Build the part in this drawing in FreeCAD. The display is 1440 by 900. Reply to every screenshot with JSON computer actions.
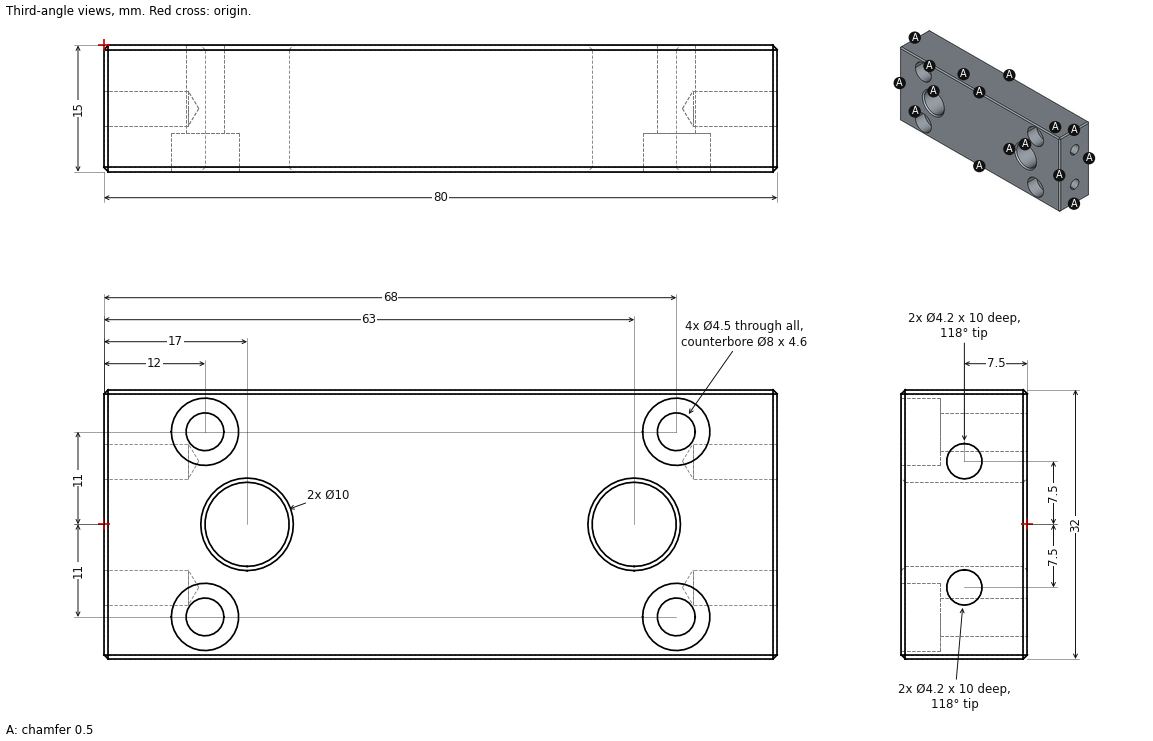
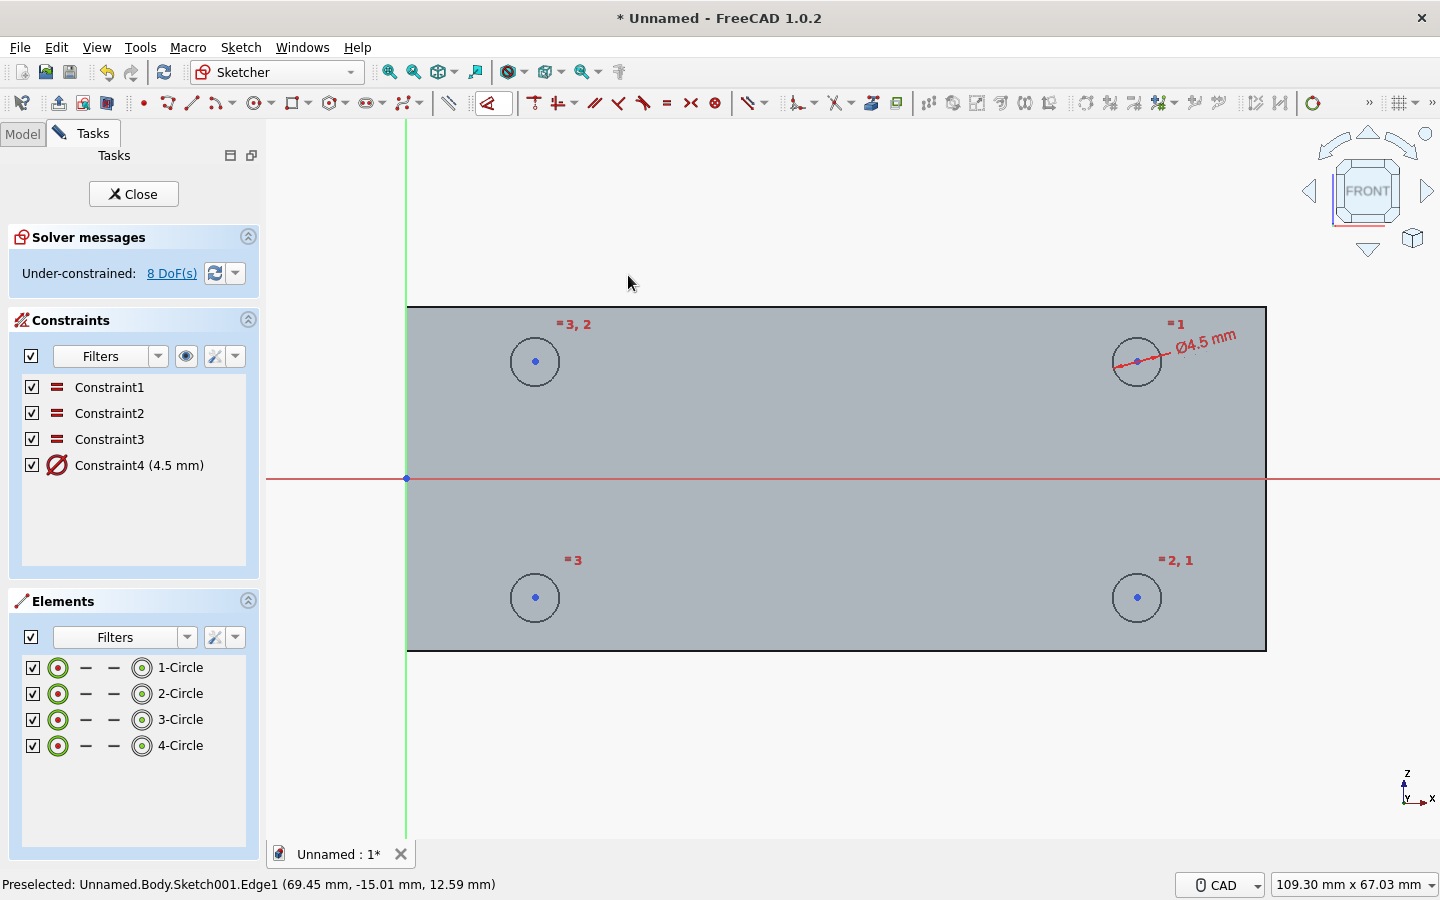
{"action": "left_click", "coordinate": [1137, 362]}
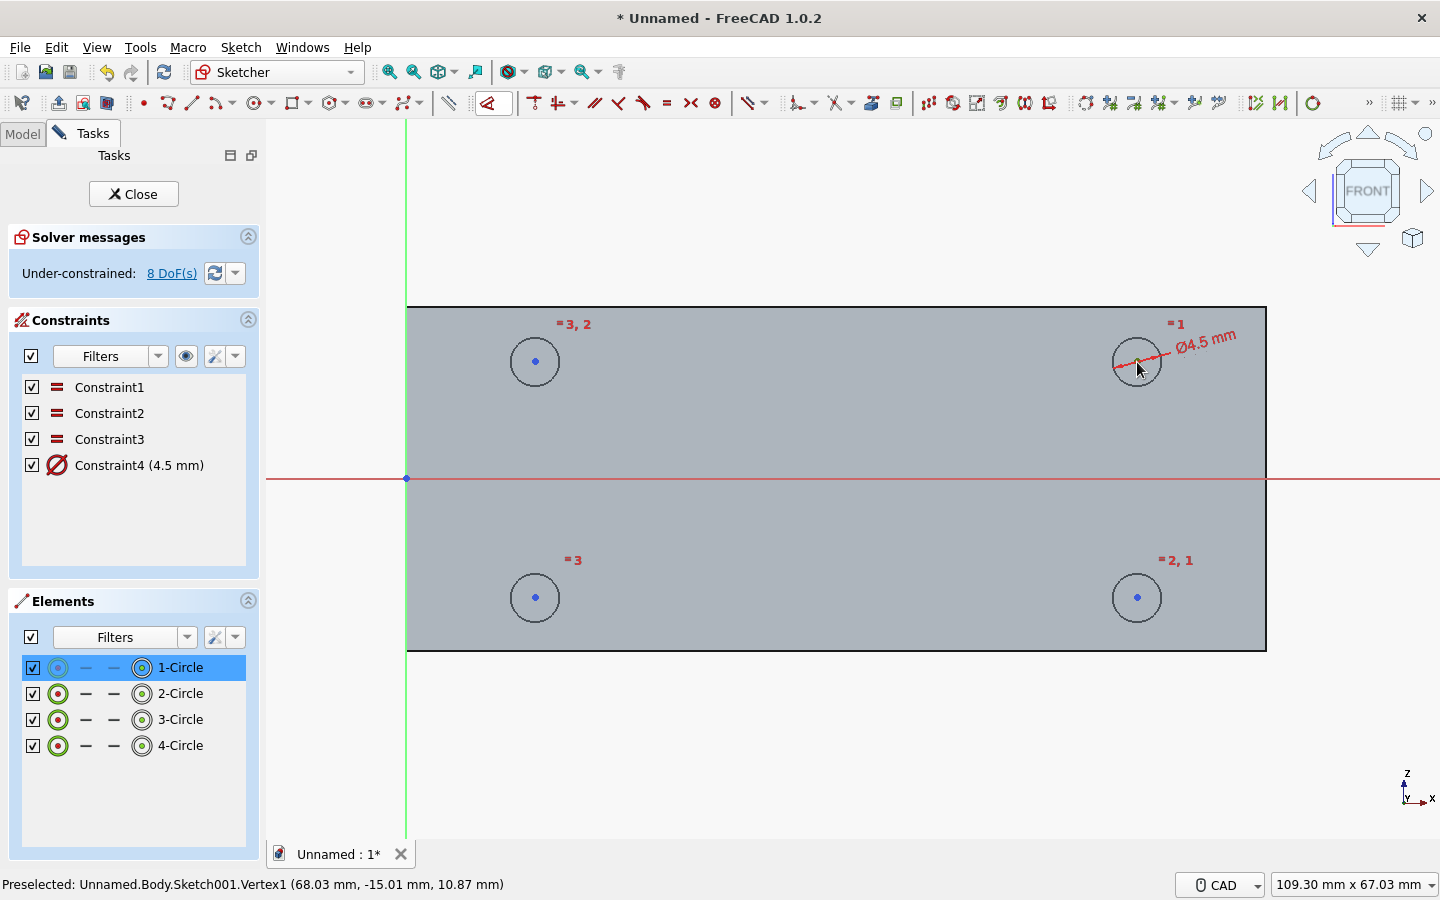
{"action": "key", "text": "l"}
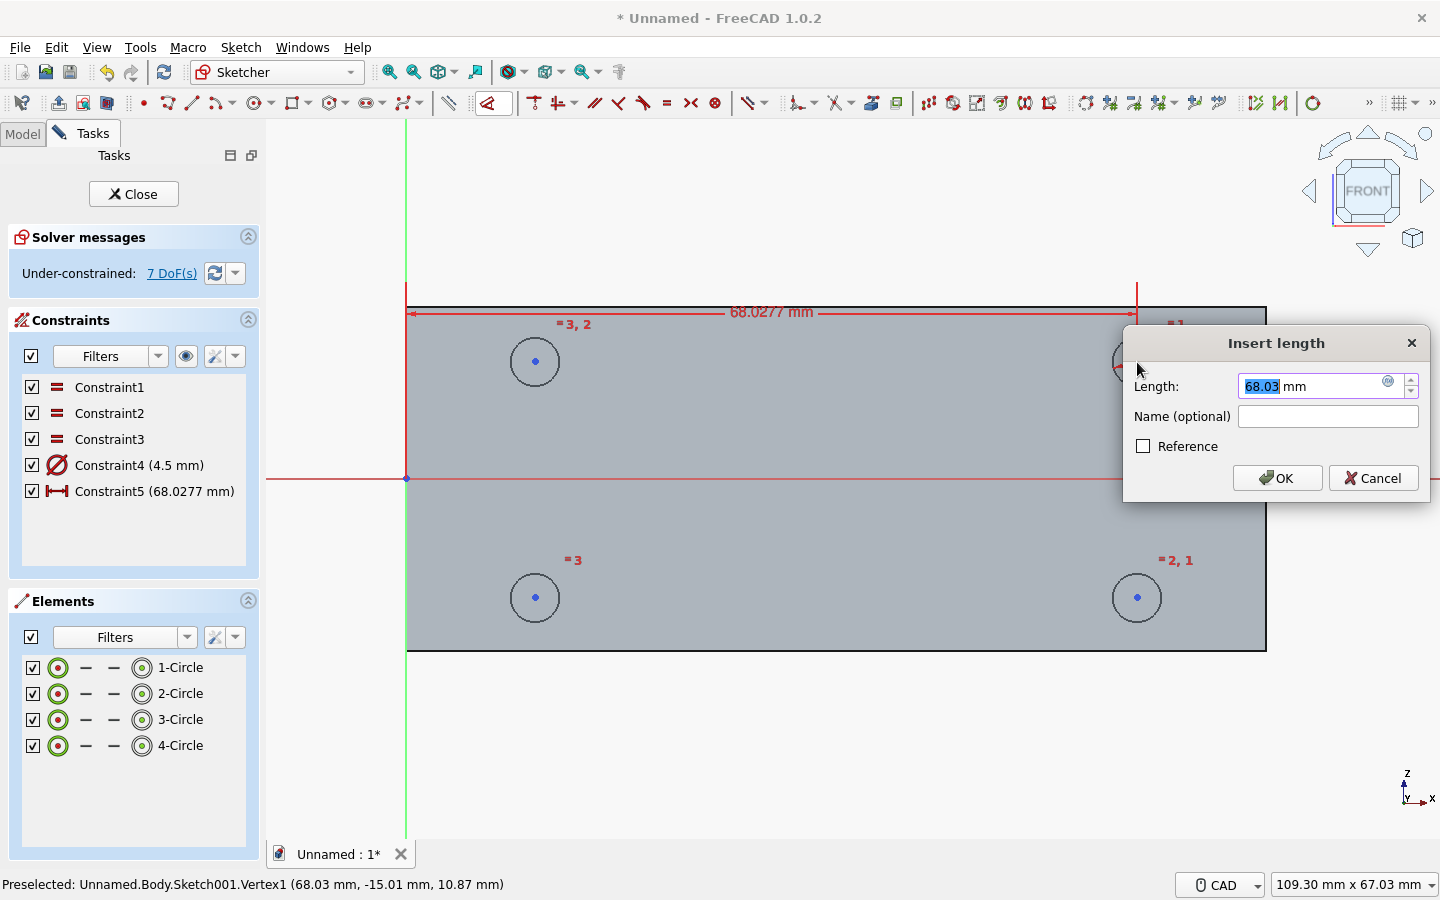
{"action": "type", "text": "68"}
{"action": "key", "text": "Return"}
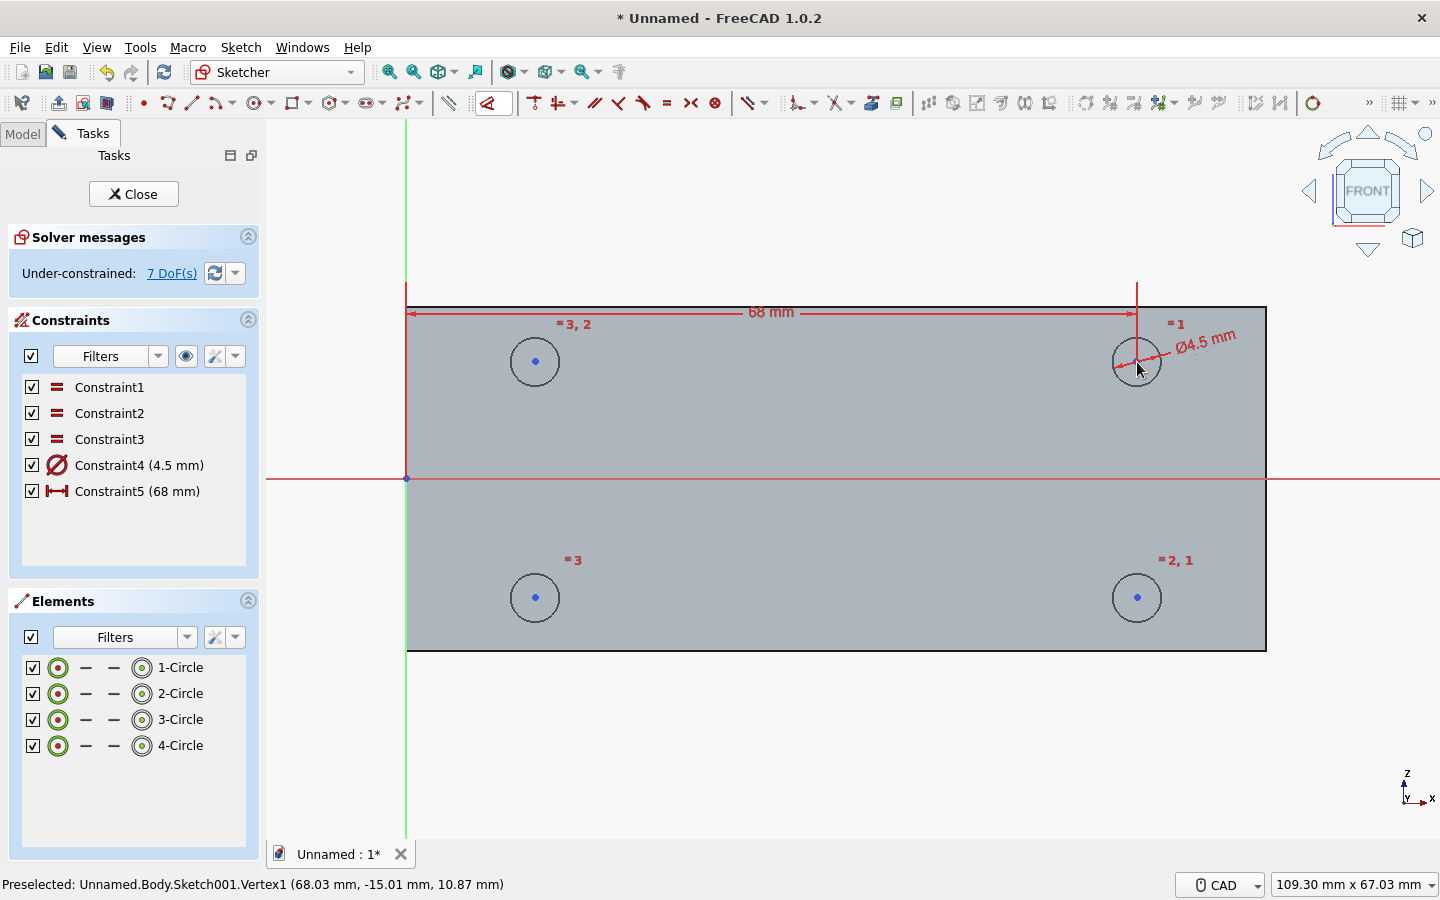
{"action": "left_click", "coordinate": [1137, 362]}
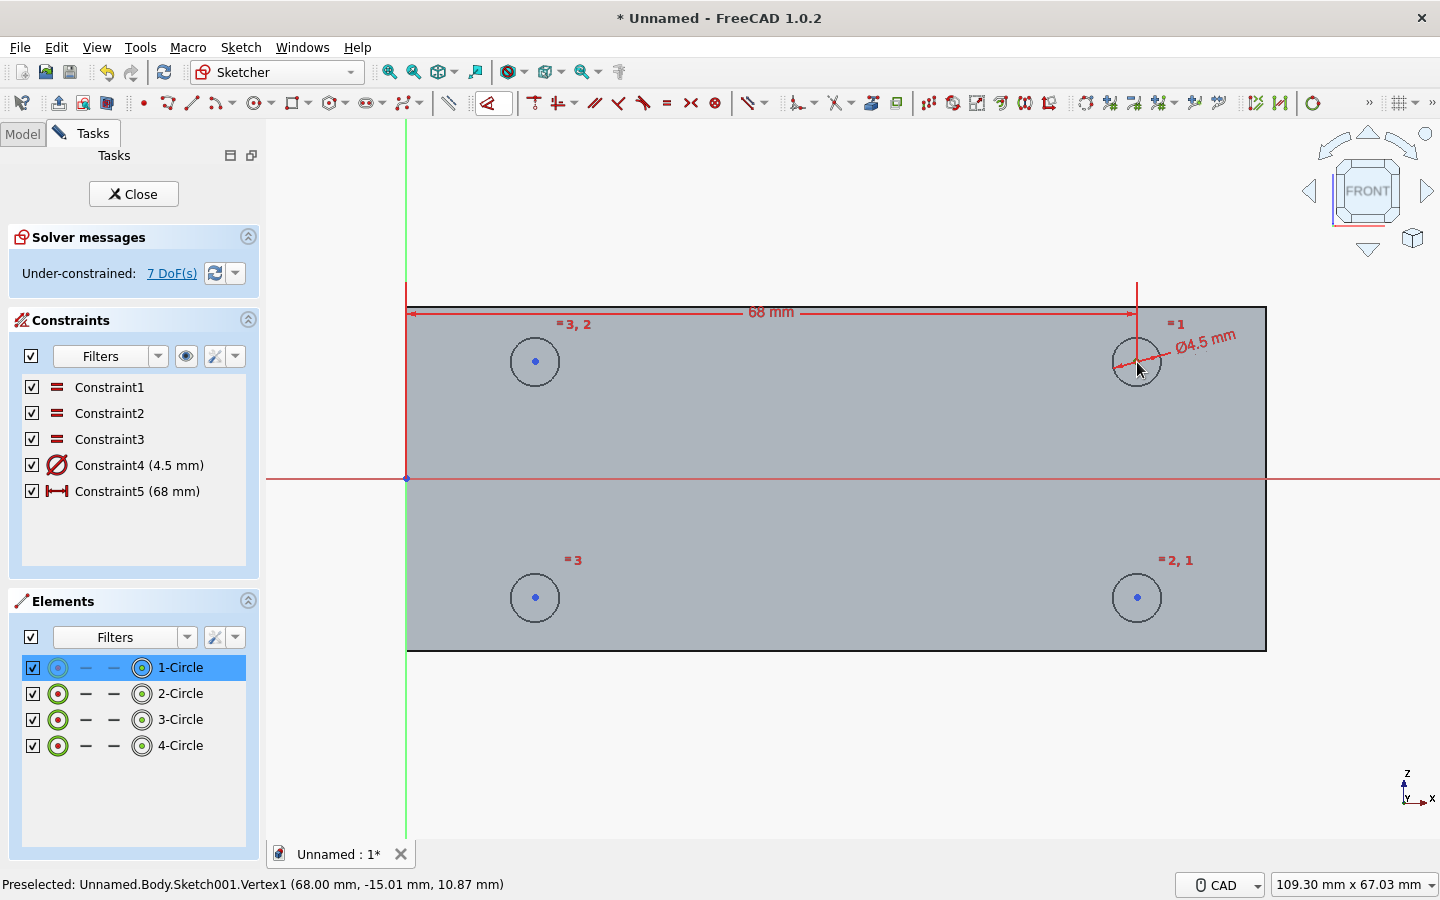
{"action": "key", "text": "i"}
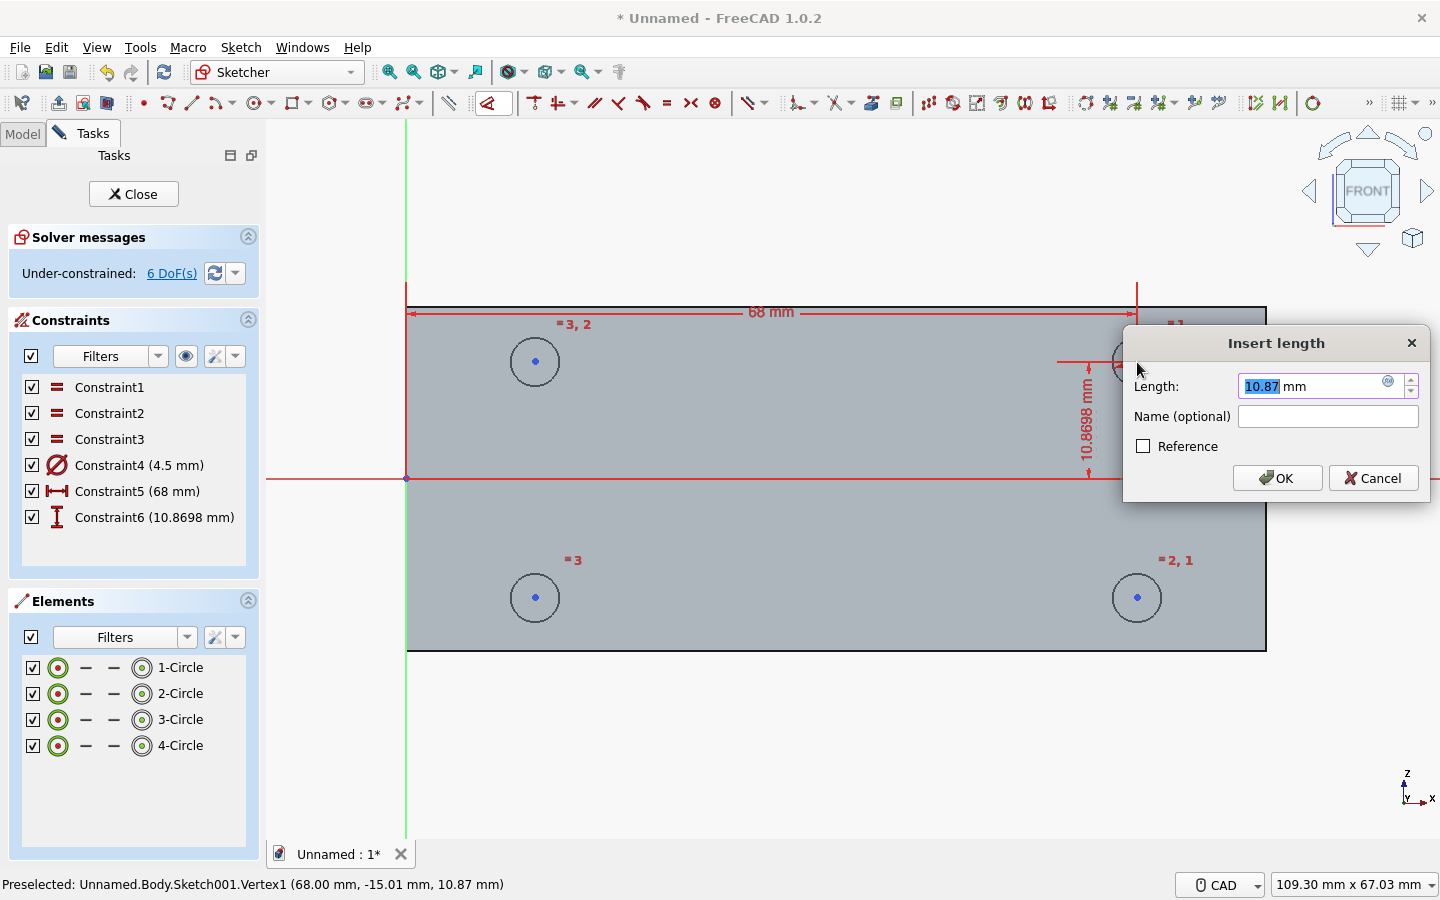
{"action": "type", "text": "11"}
{"action": "key", "text": "Return"}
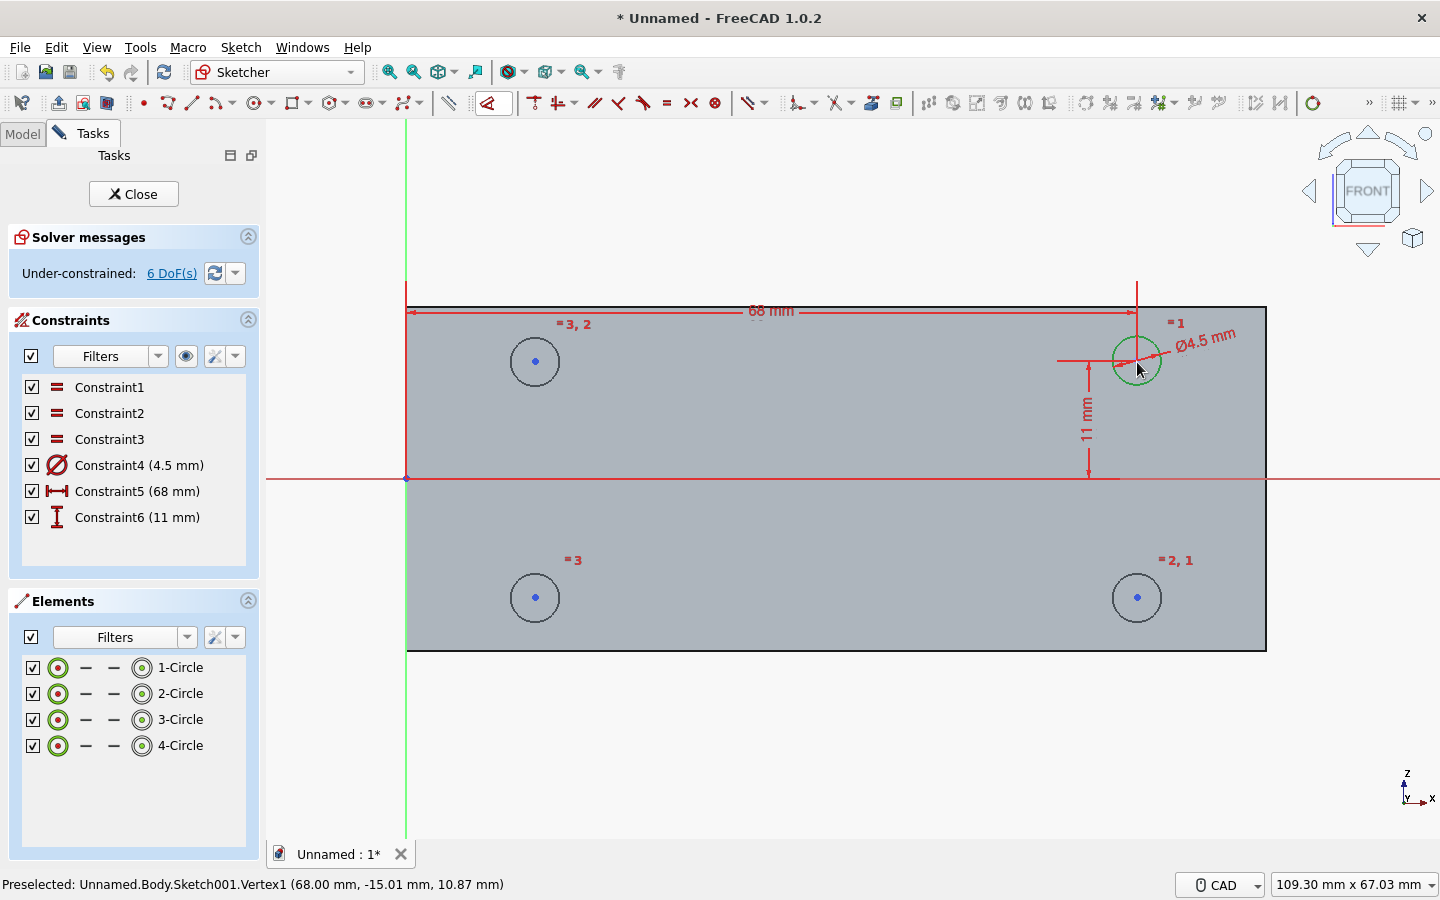
{"action": "left_click", "coordinate": [1137, 598]}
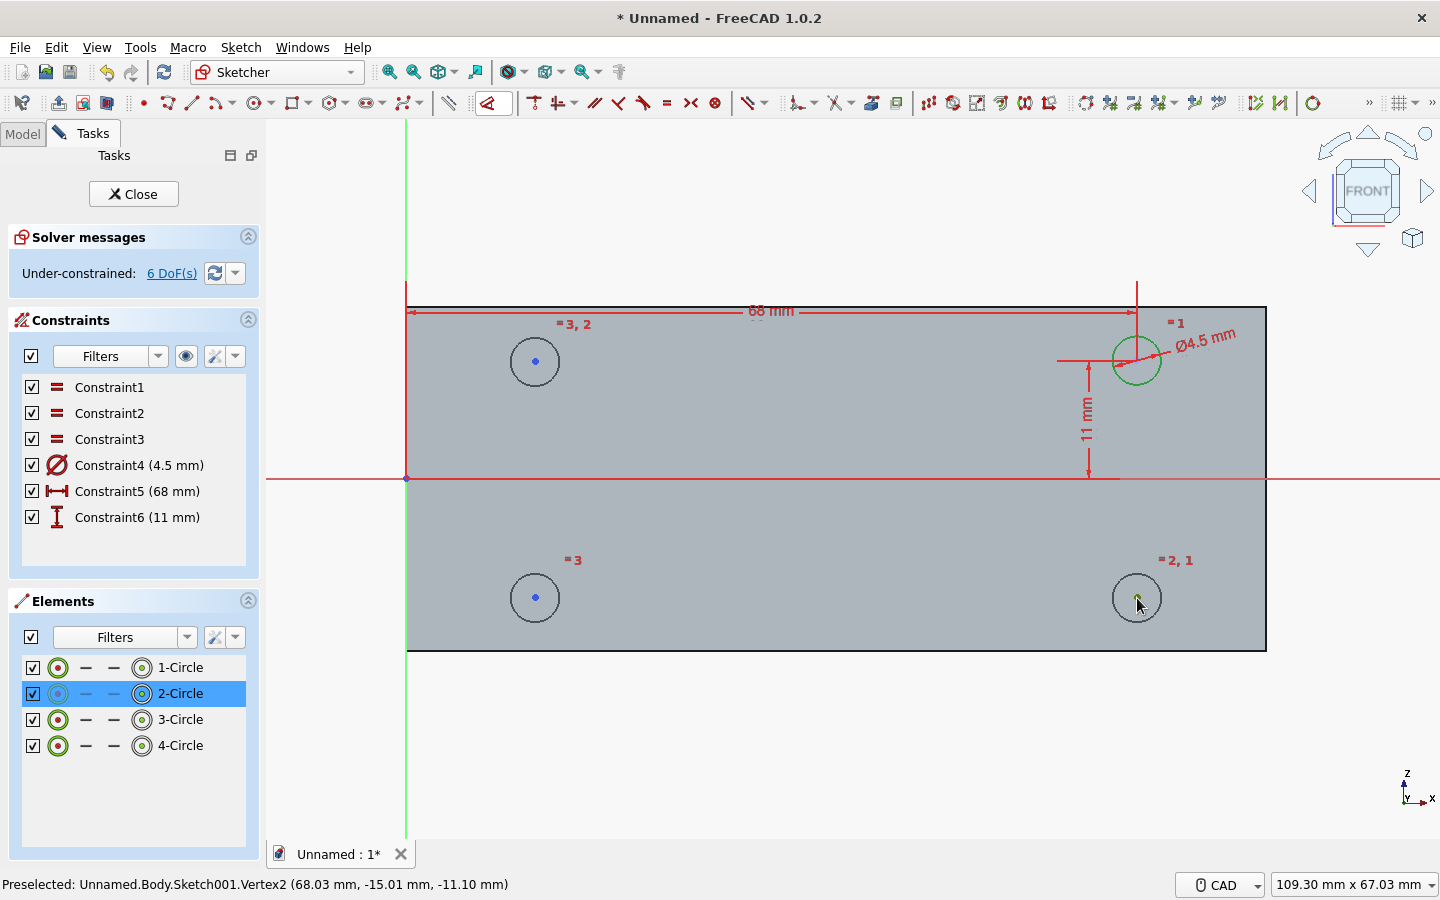
{"action": "left_click", "coordinate": [506, 104]}